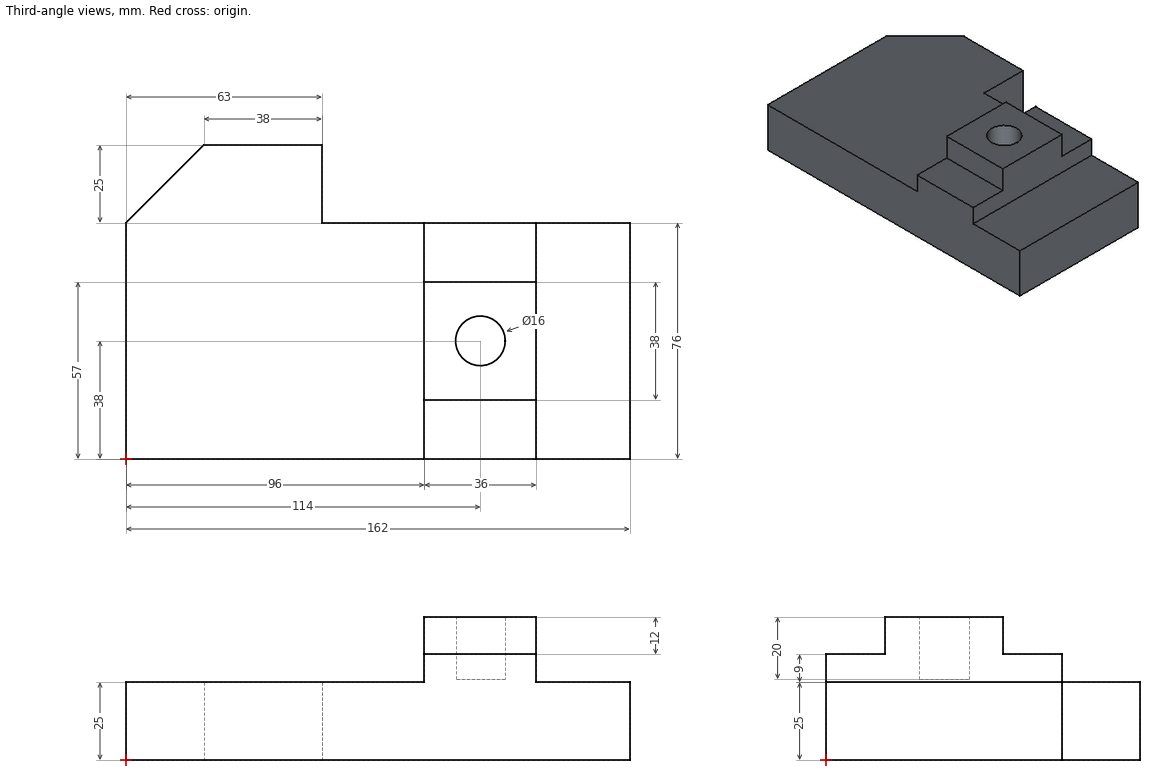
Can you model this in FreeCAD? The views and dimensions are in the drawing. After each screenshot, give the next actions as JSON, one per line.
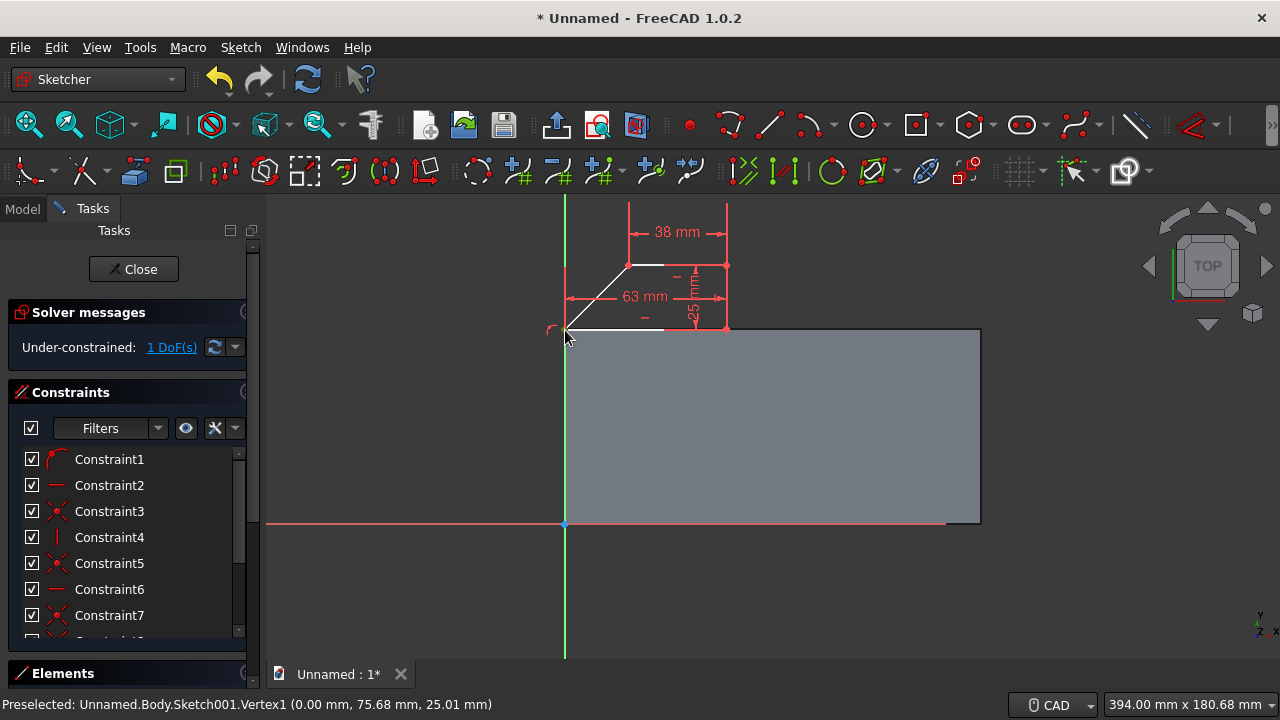
{"action": "left_click", "coordinate": [1218, 126]}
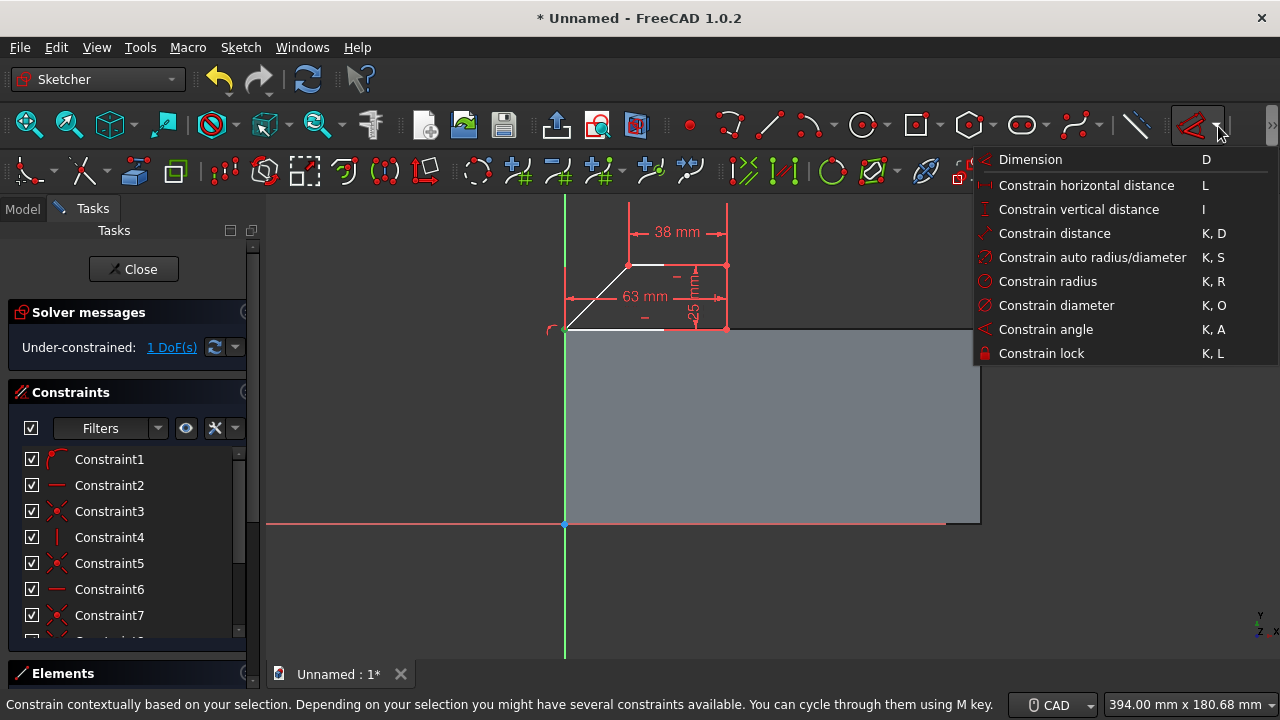
{"action": "left_click", "coordinate": [1126, 209]}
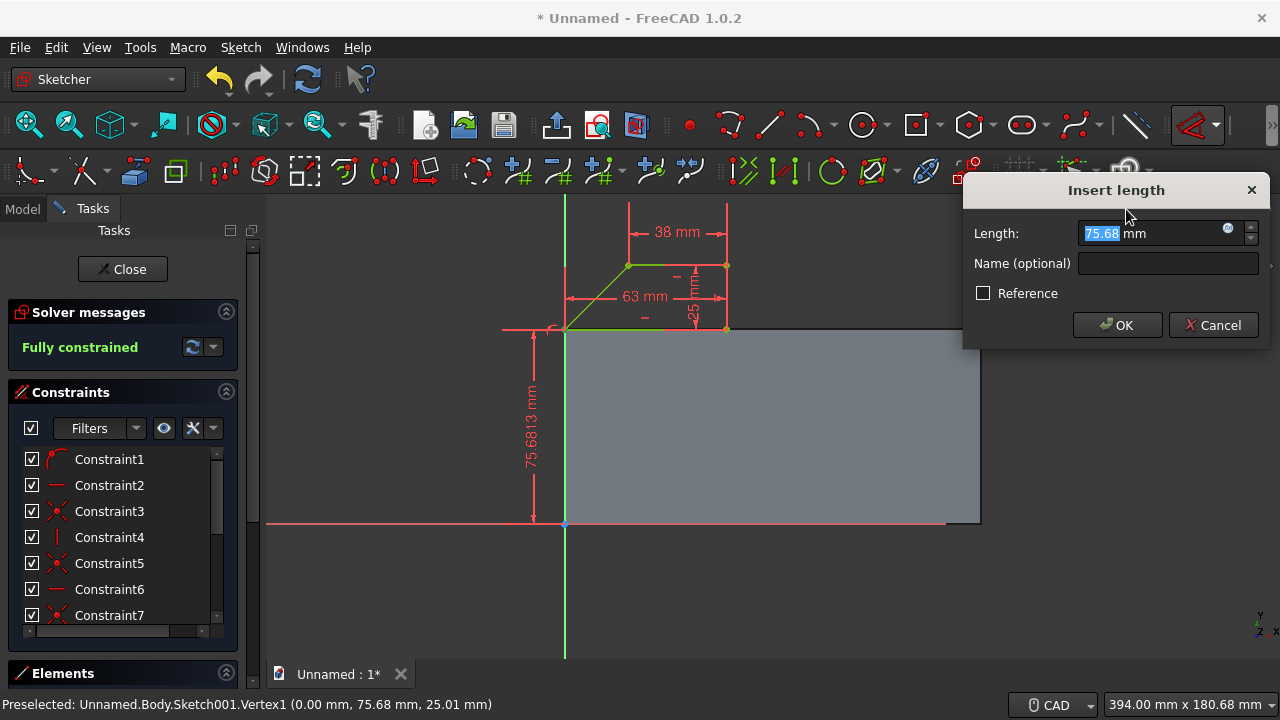
{"action": "type", "text": "76"}
{"action": "key", "text": "Return"}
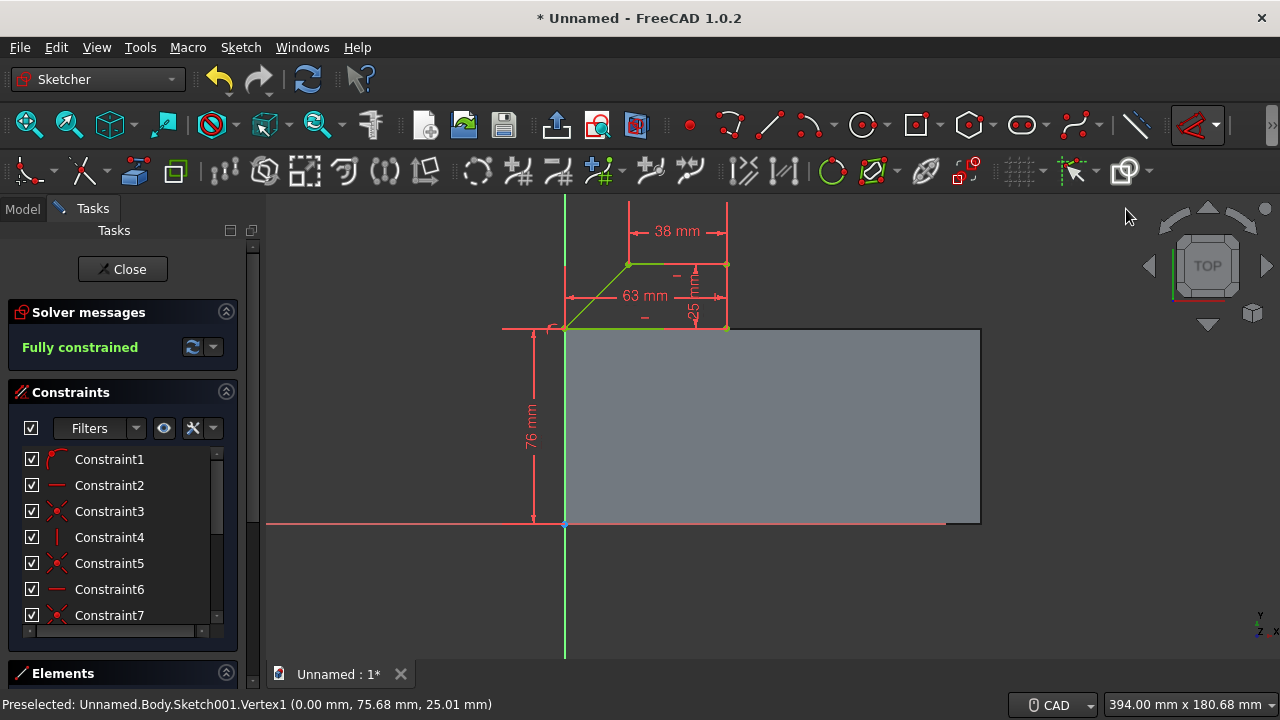
{"action": "left_click", "coordinate": [123, 269]}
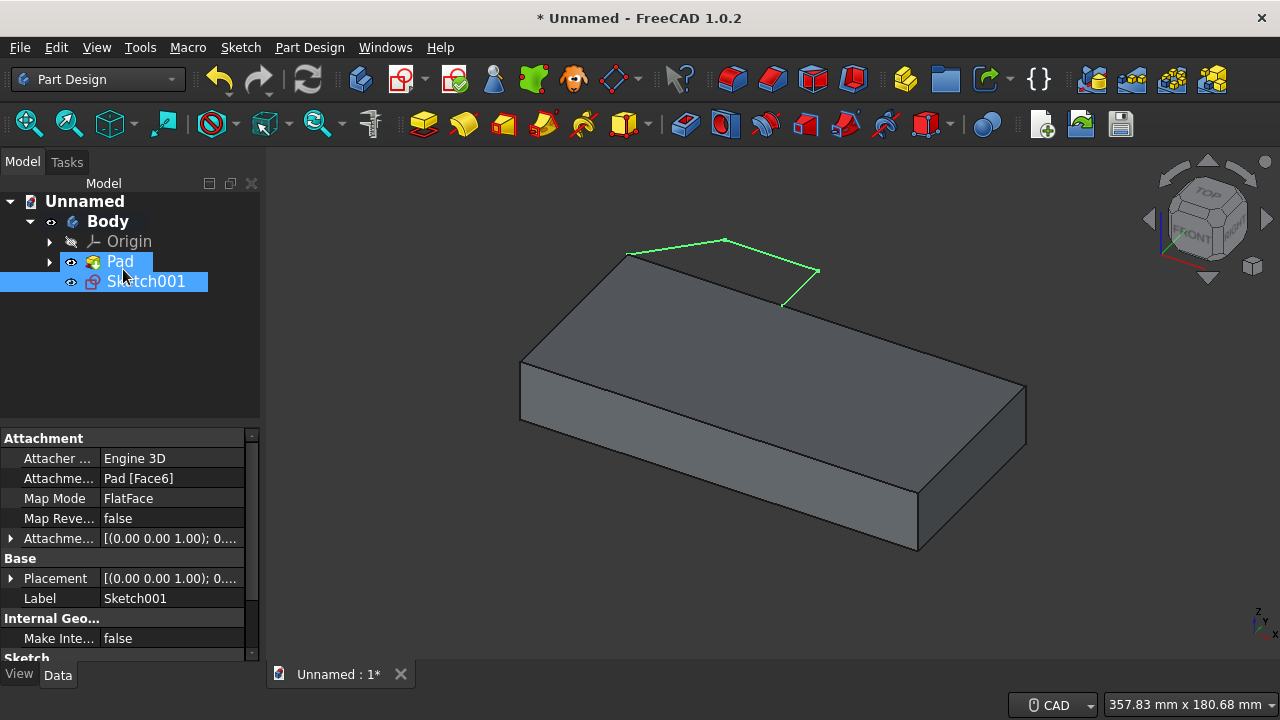
{"action": "left_click", "coordinate": [424, 124]}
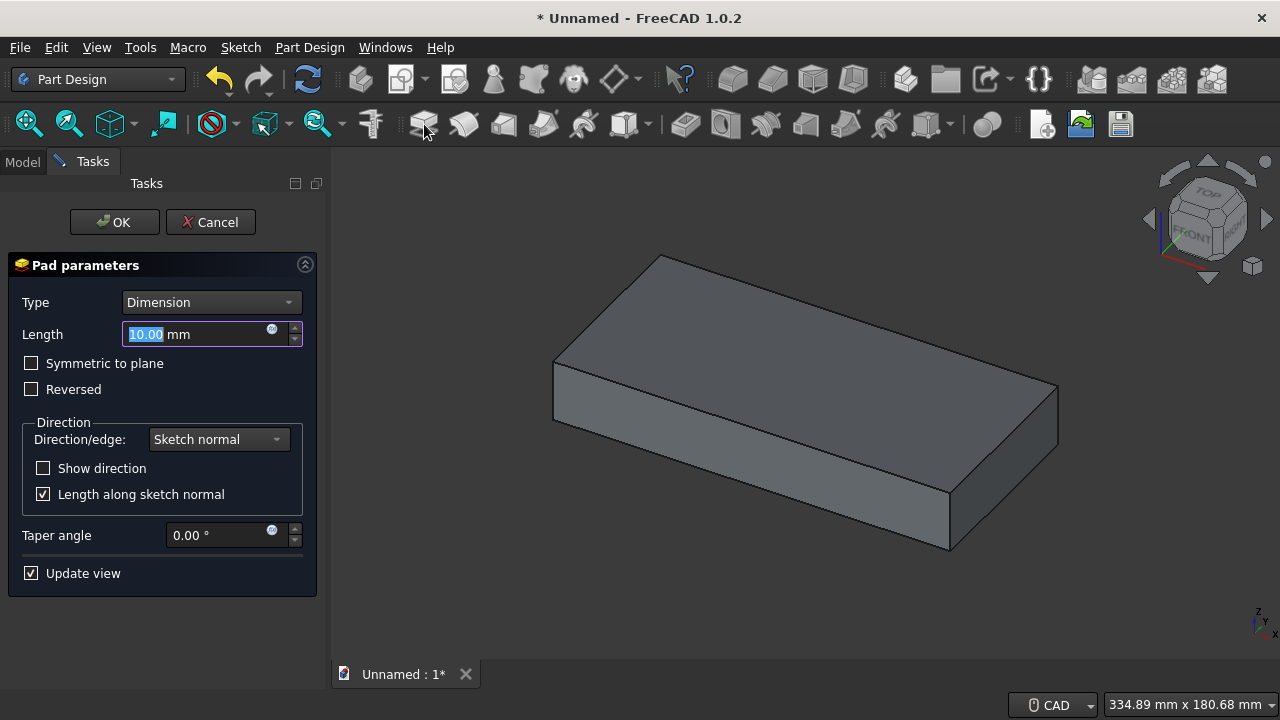
{"action": "type", "text": "25"}
{"action": "key", "text": "Tab"}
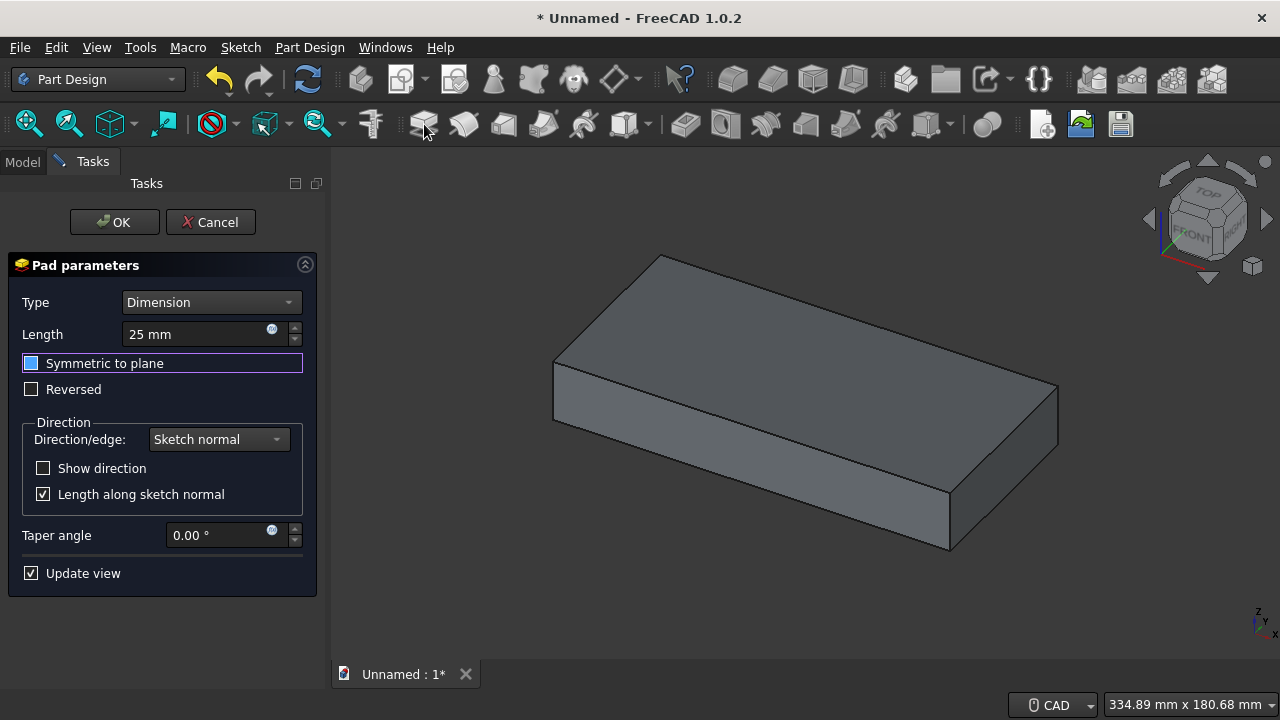
{"action": "left_click", "coordinate": [30, 389]}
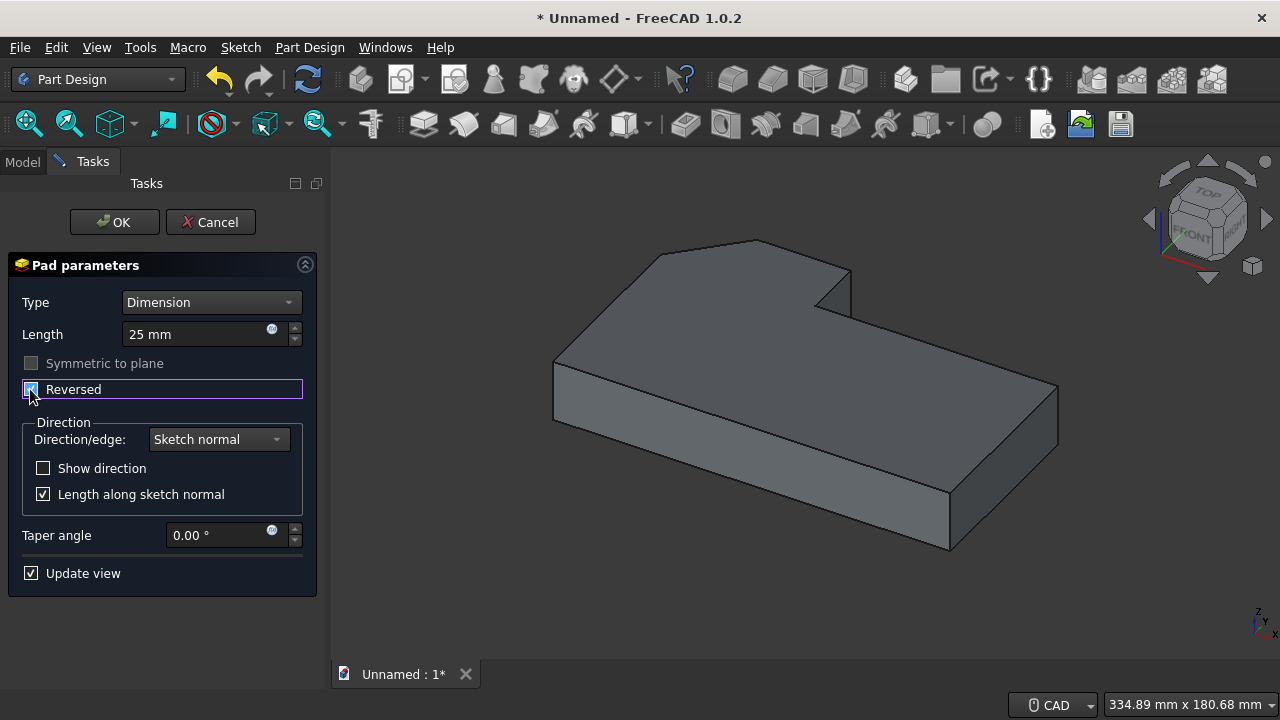
{"action": "left_click", "coordinate": [115, 222]}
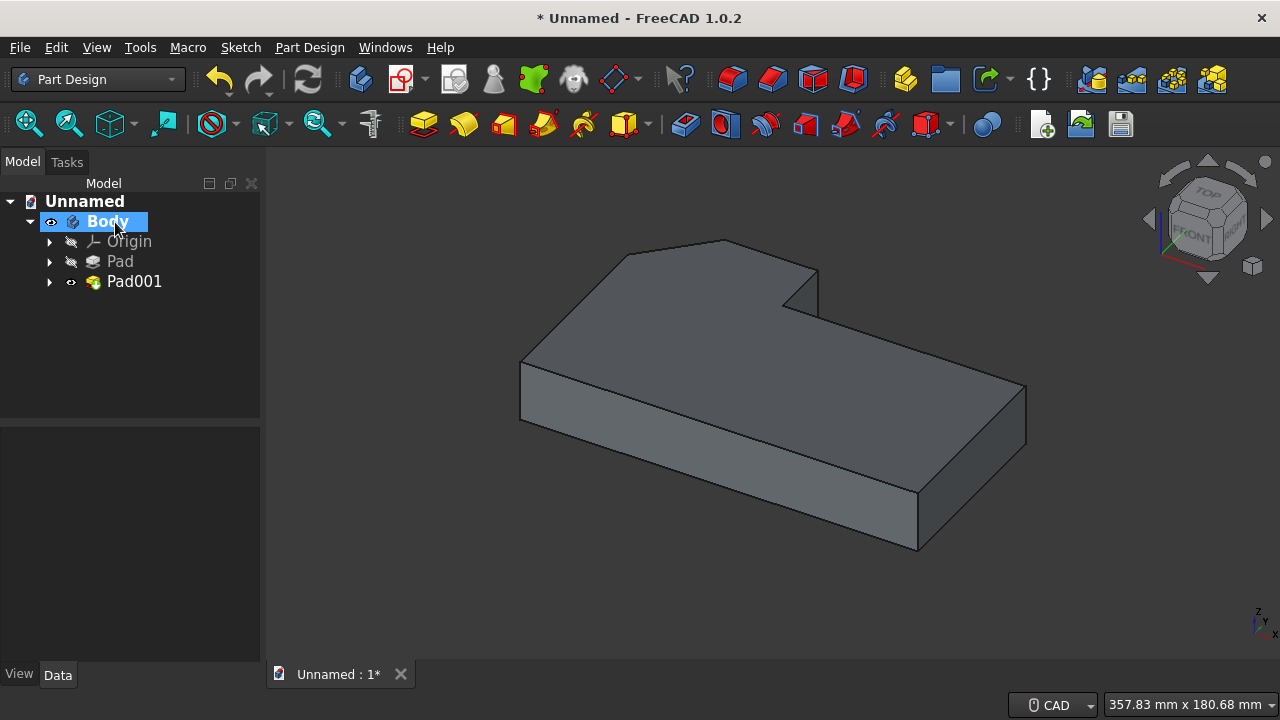
{"action": "left_click", "coordinate": [827, 395]}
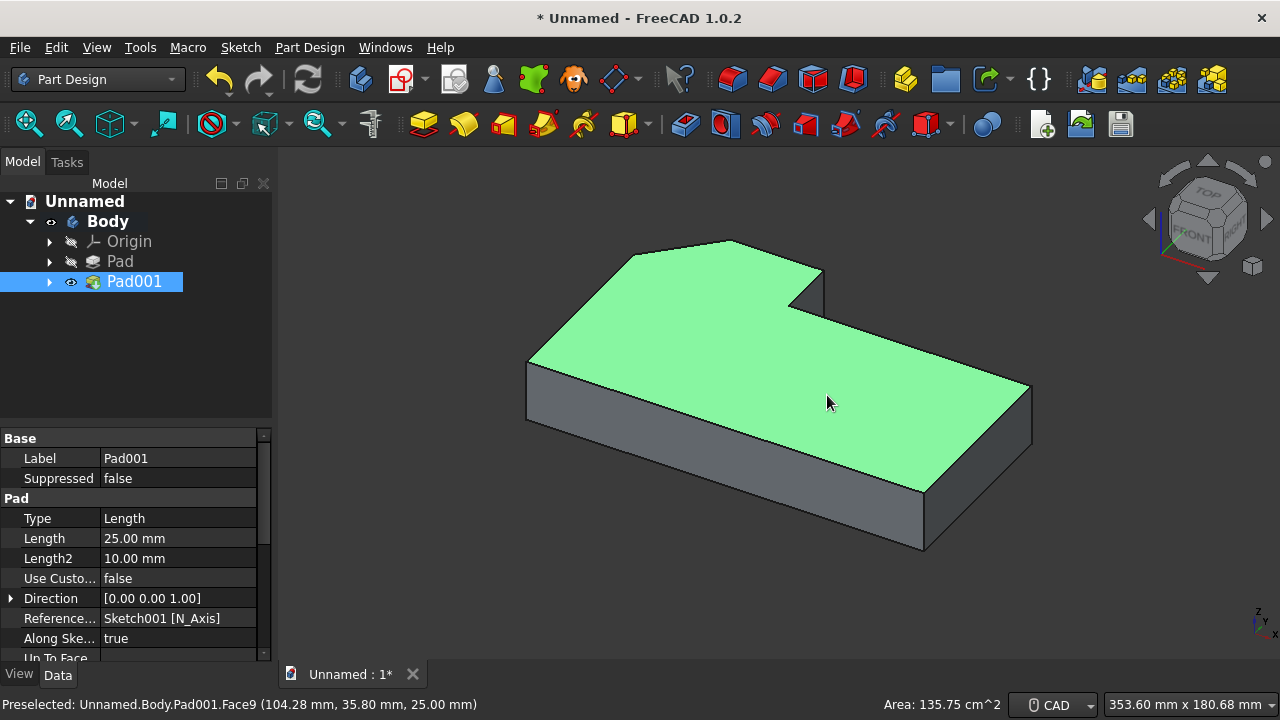
{"action": "left_click", "coordinate": [402, 80]}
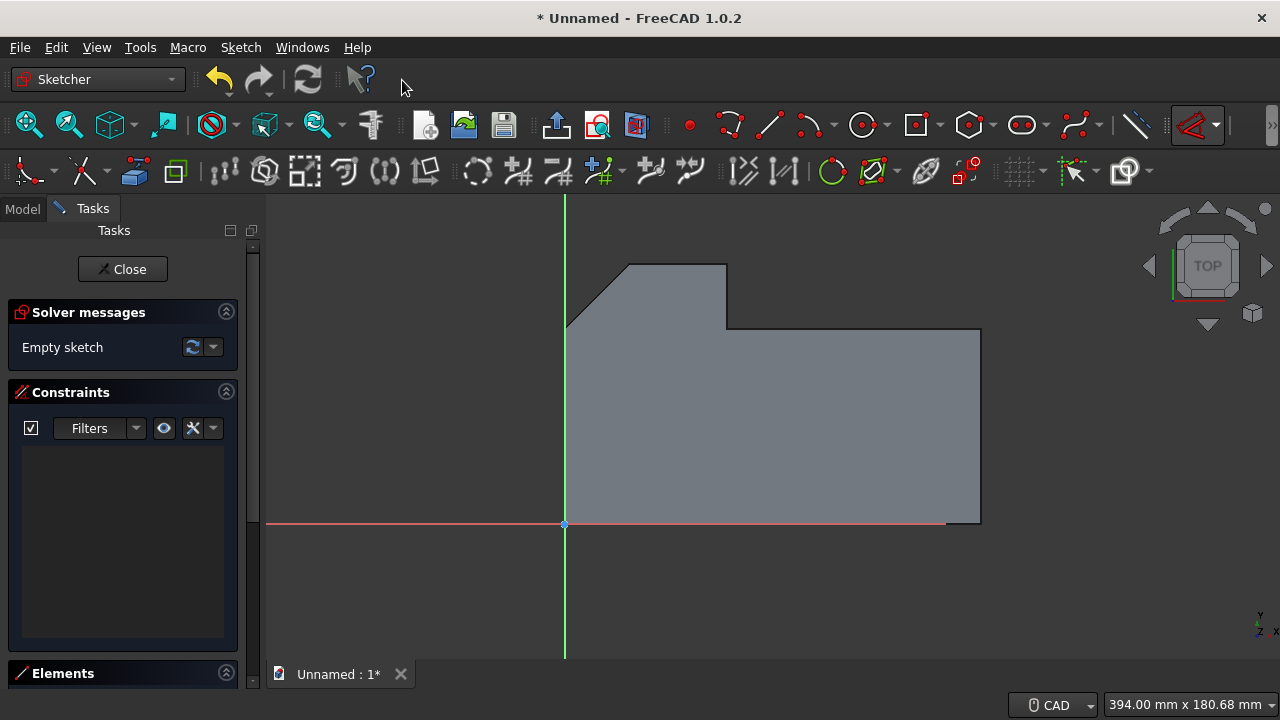
{"action": "scroll", "coordinate": [795, 426], "scroll_direction": "up", "scroll_amount": 2}